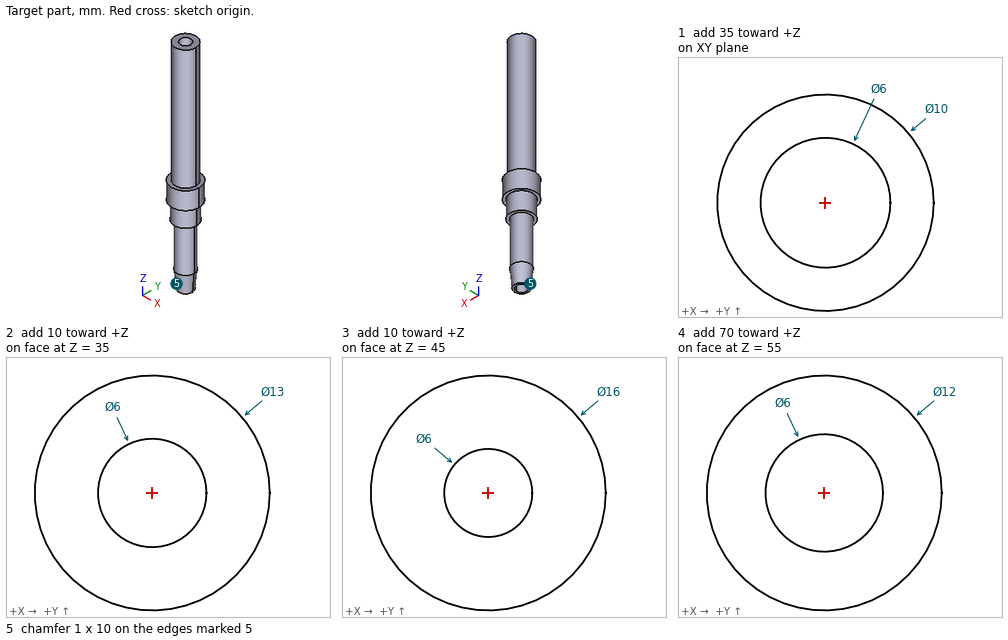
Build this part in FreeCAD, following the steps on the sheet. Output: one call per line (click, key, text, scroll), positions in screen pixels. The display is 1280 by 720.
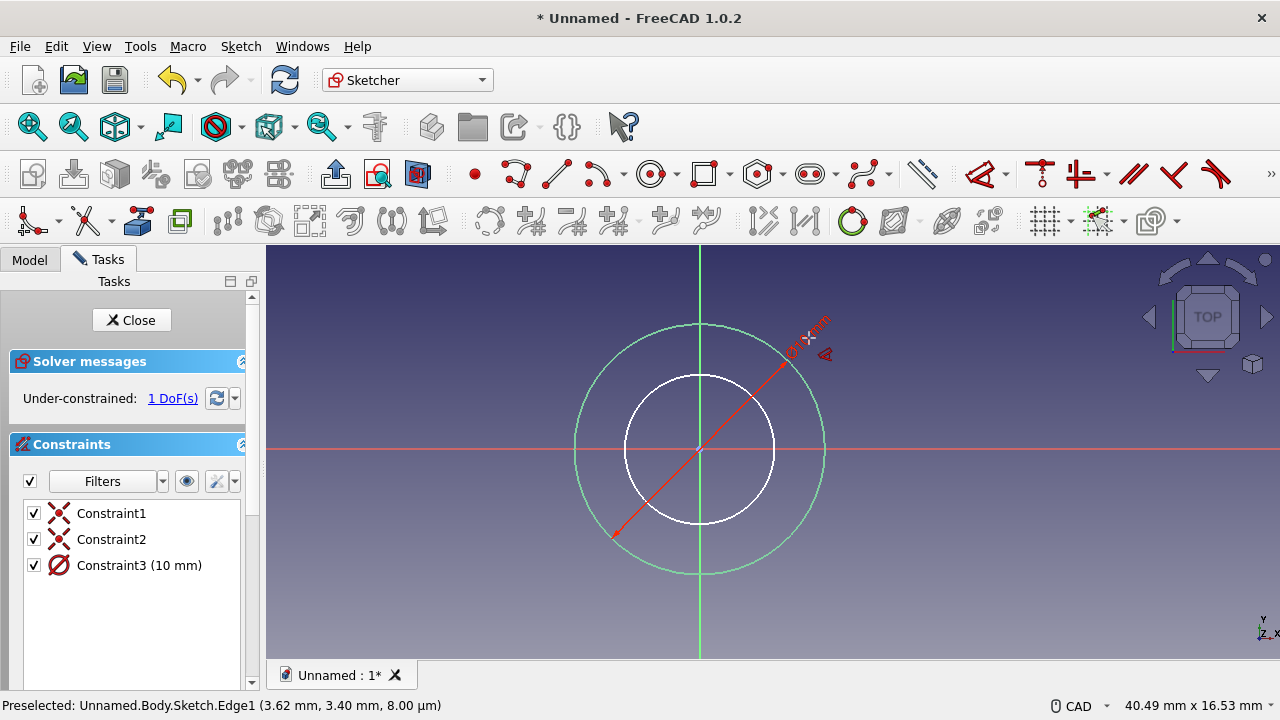
click(752, 396)
click(774, 373)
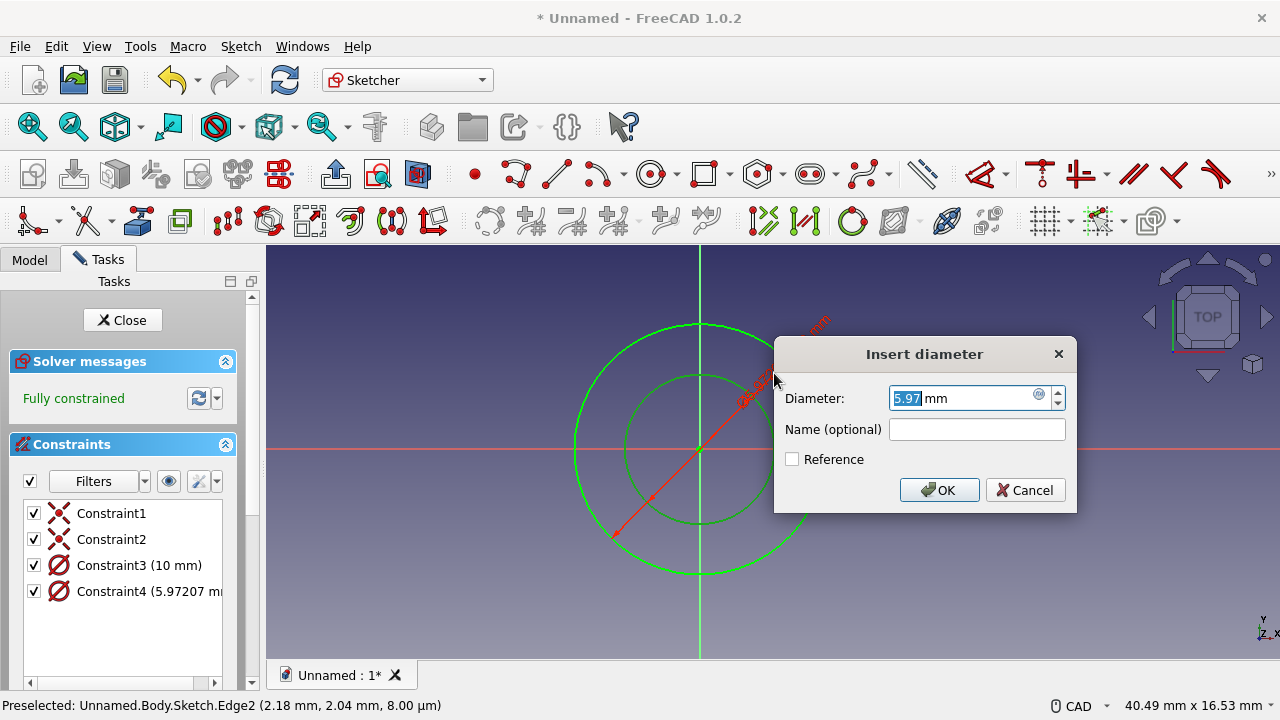
text(6)
key(Return)
key(Escape)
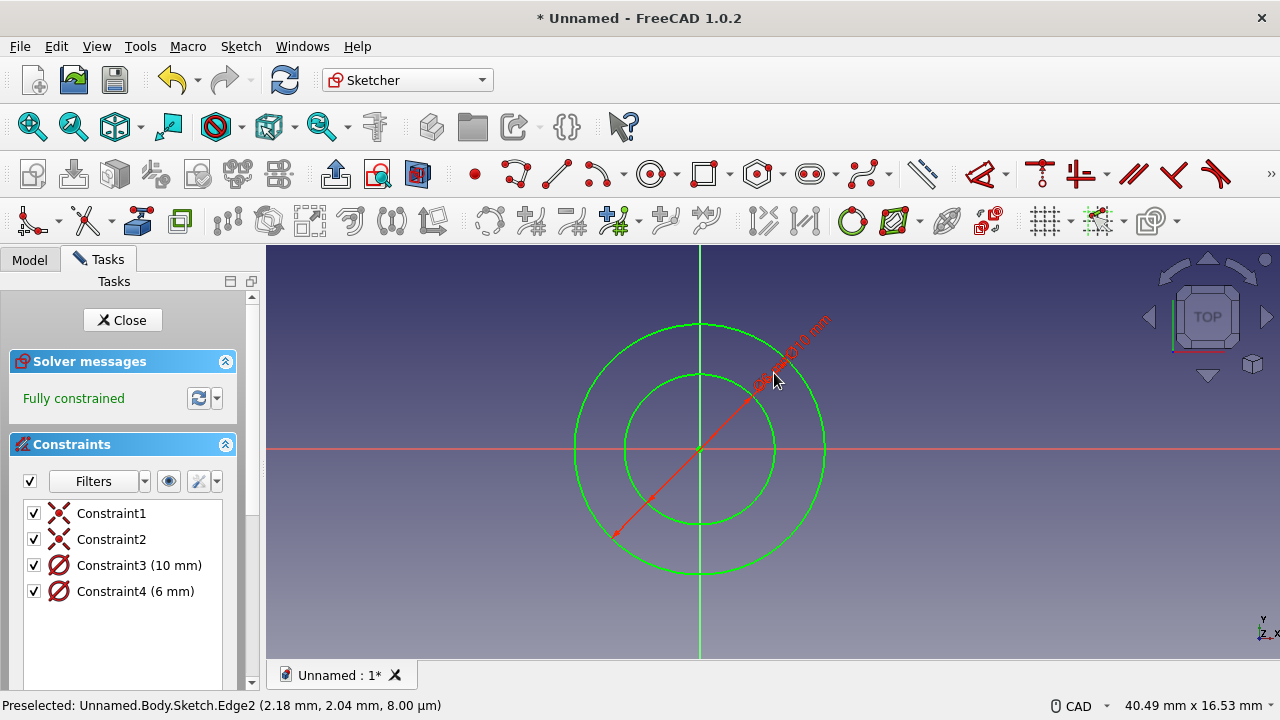
click(123, 320)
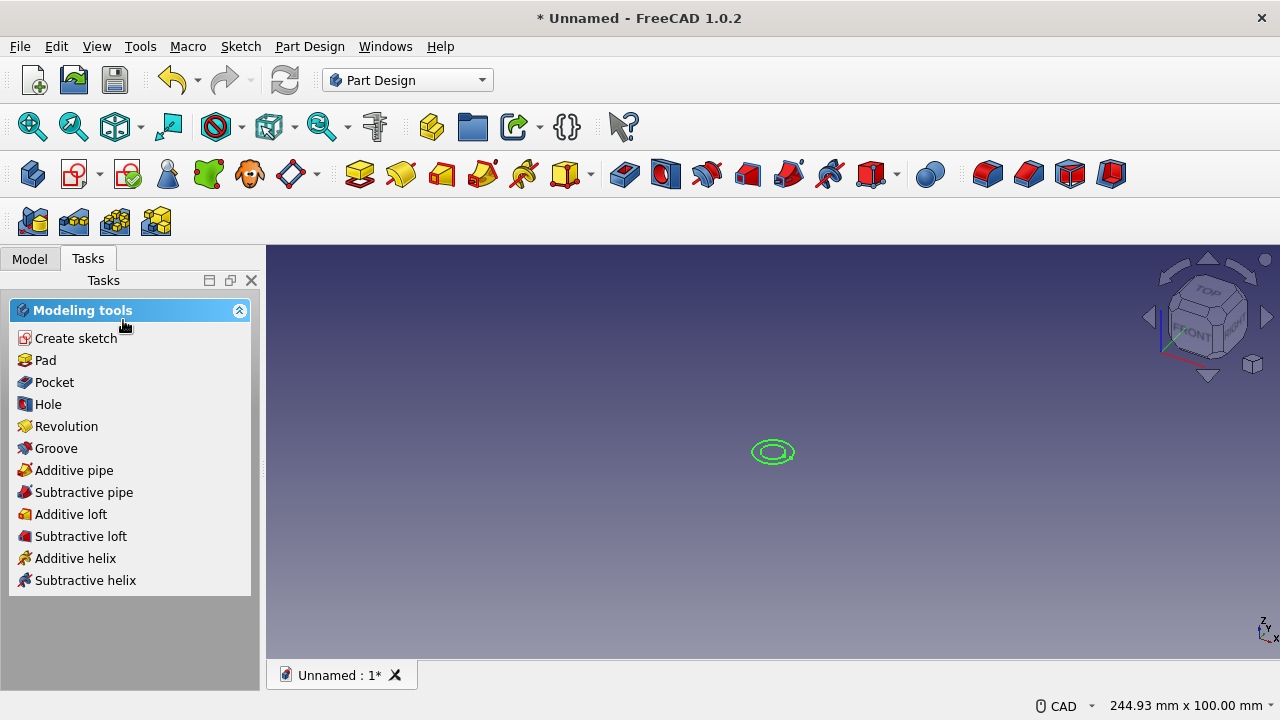
click(360, 174)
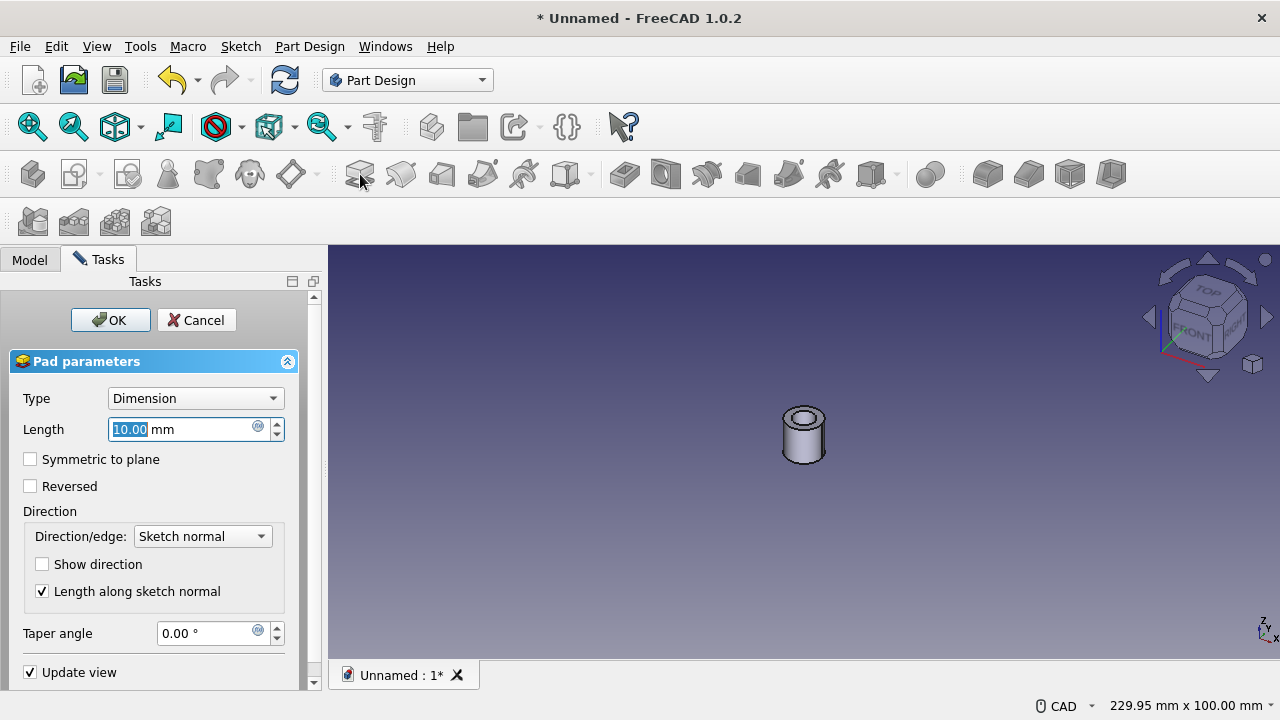
text(35)
key(Tab)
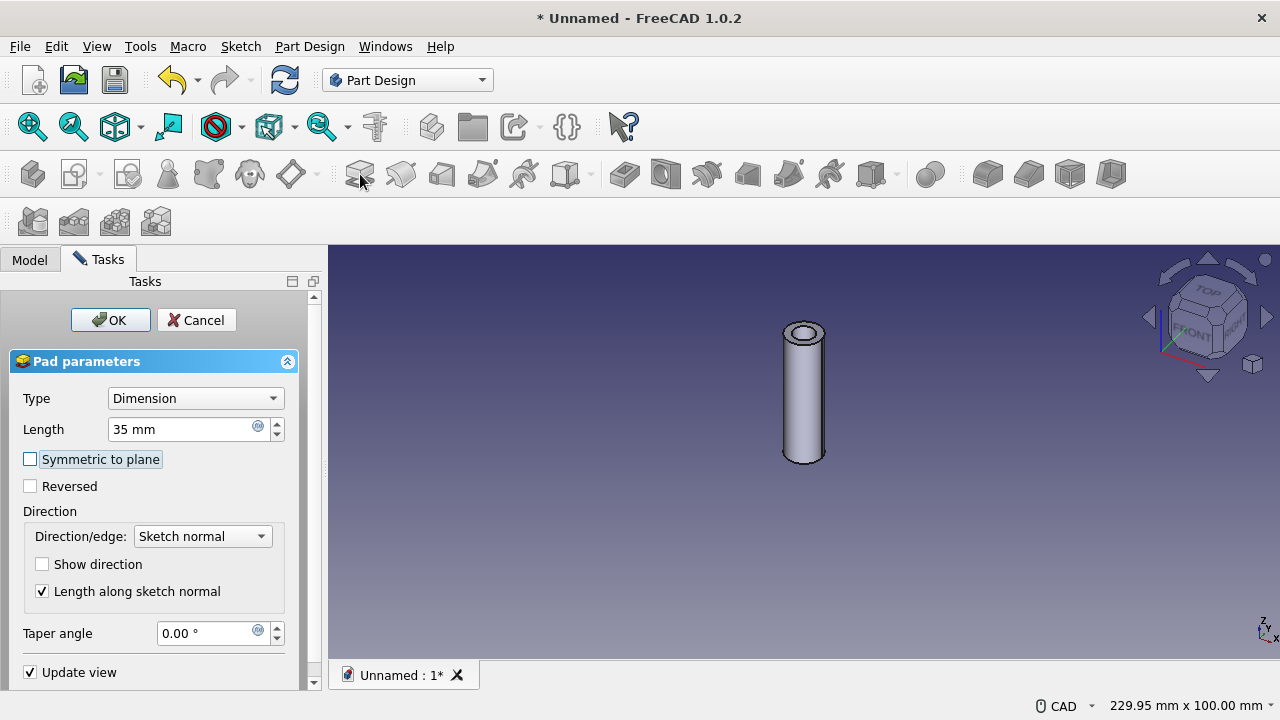
click(111, 320)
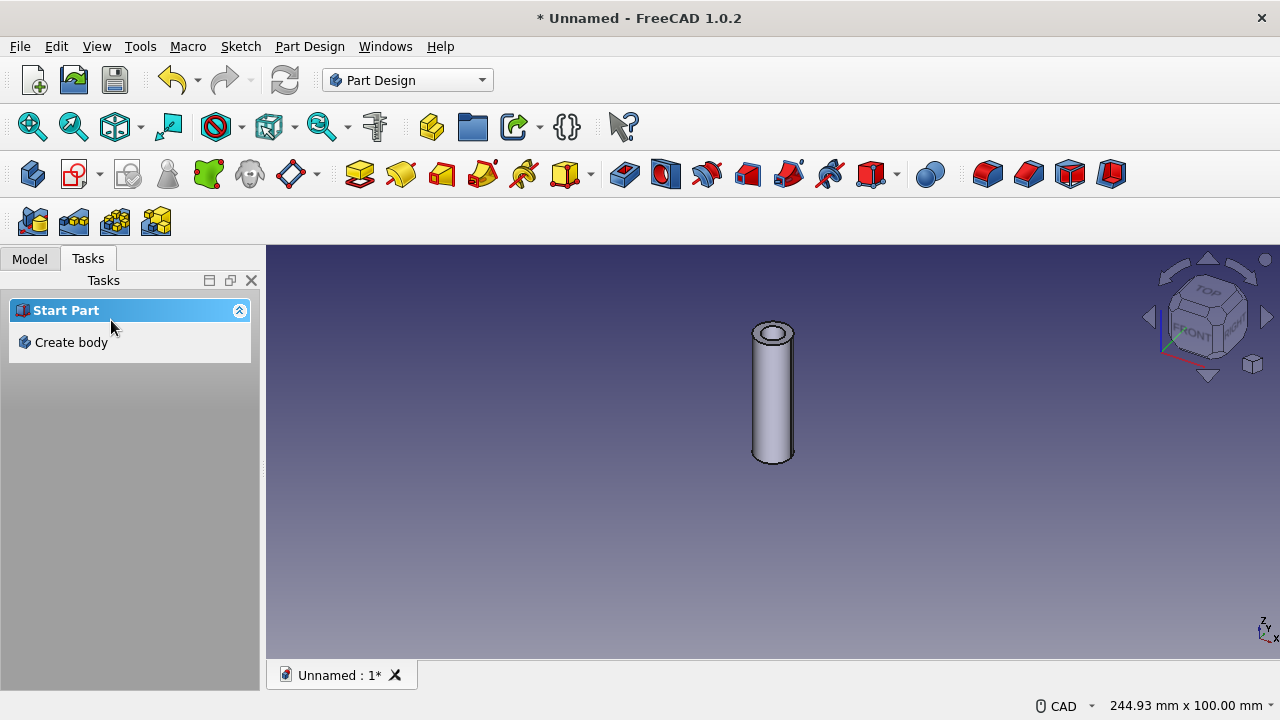
click(33, 128)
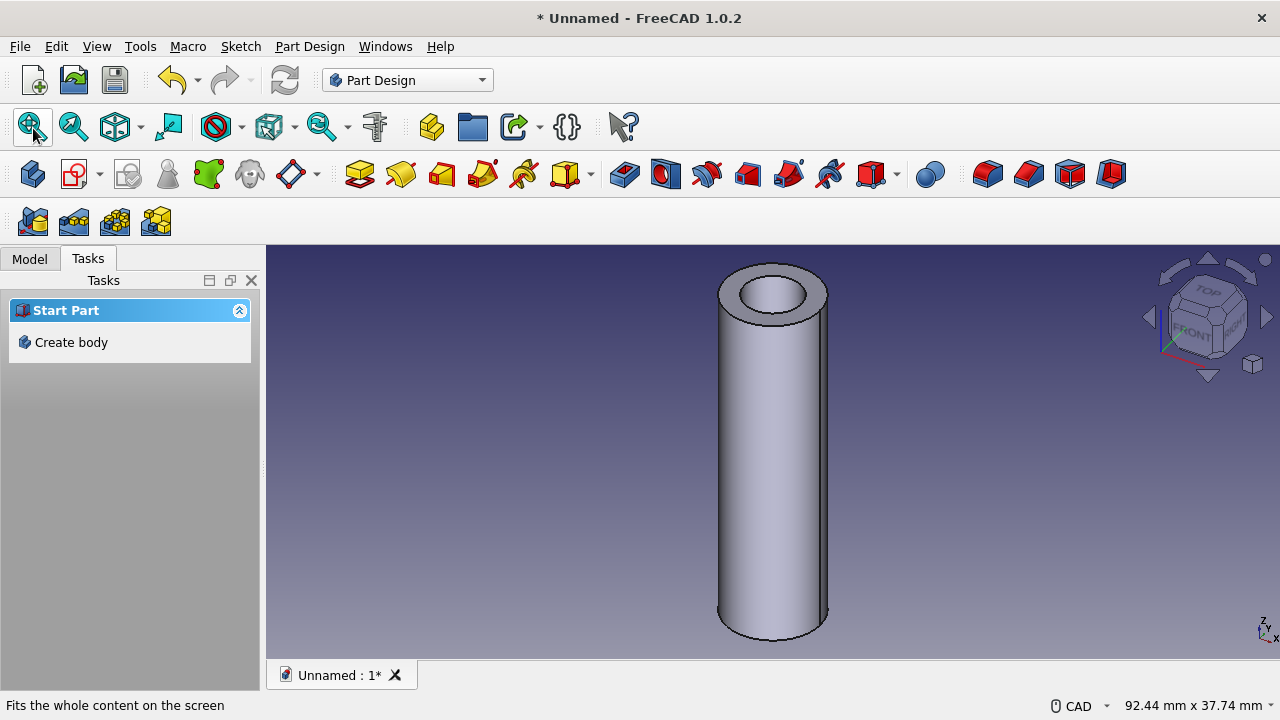
click(816, 287)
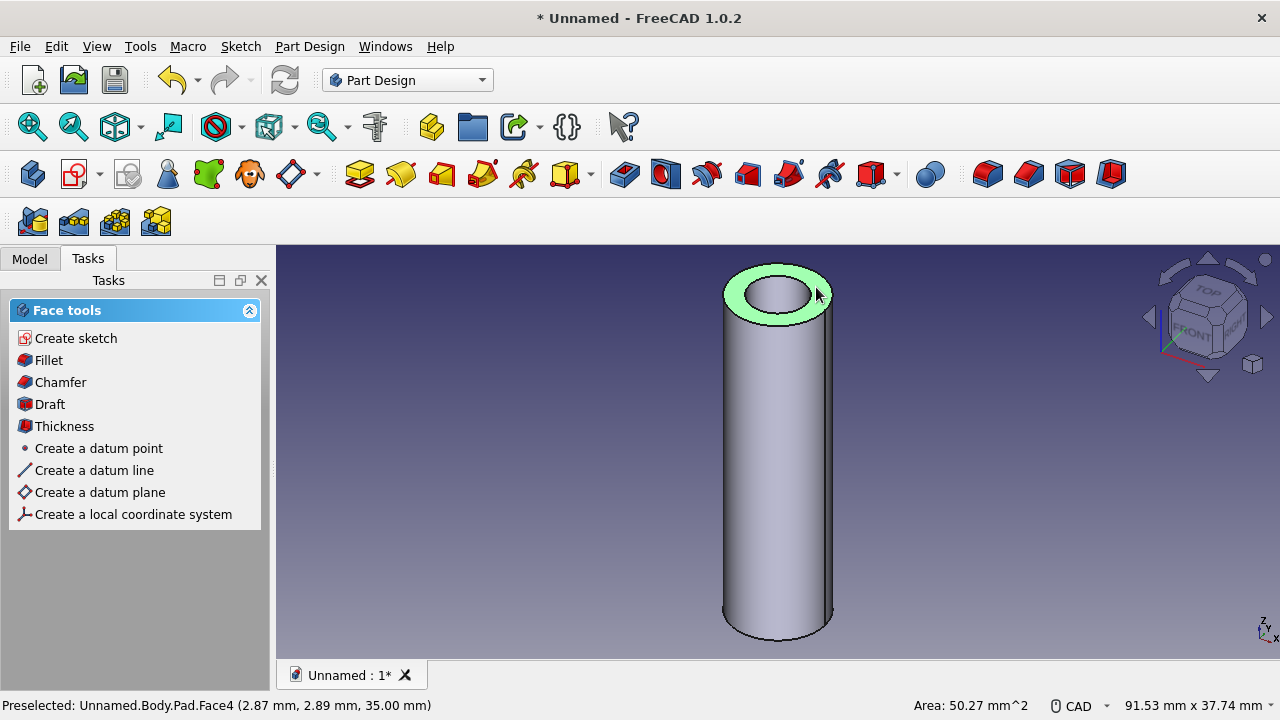
click(74, 174)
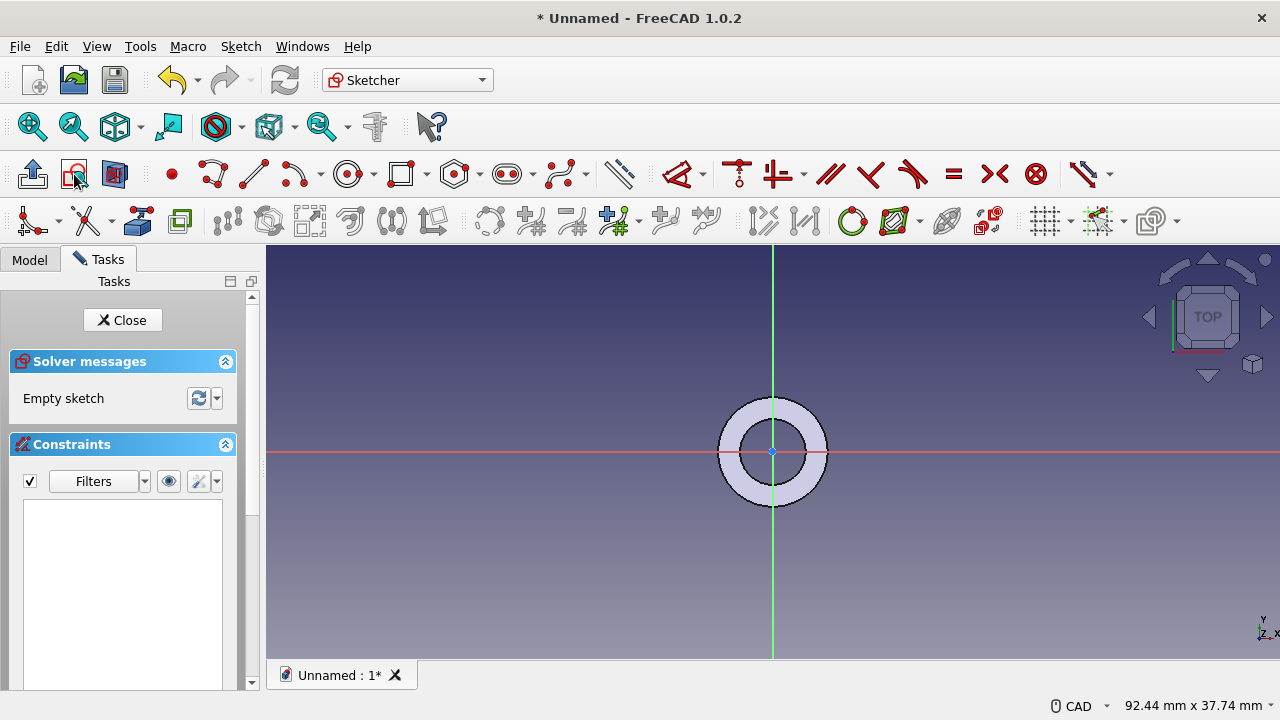
scroll(856, 452, up, 3)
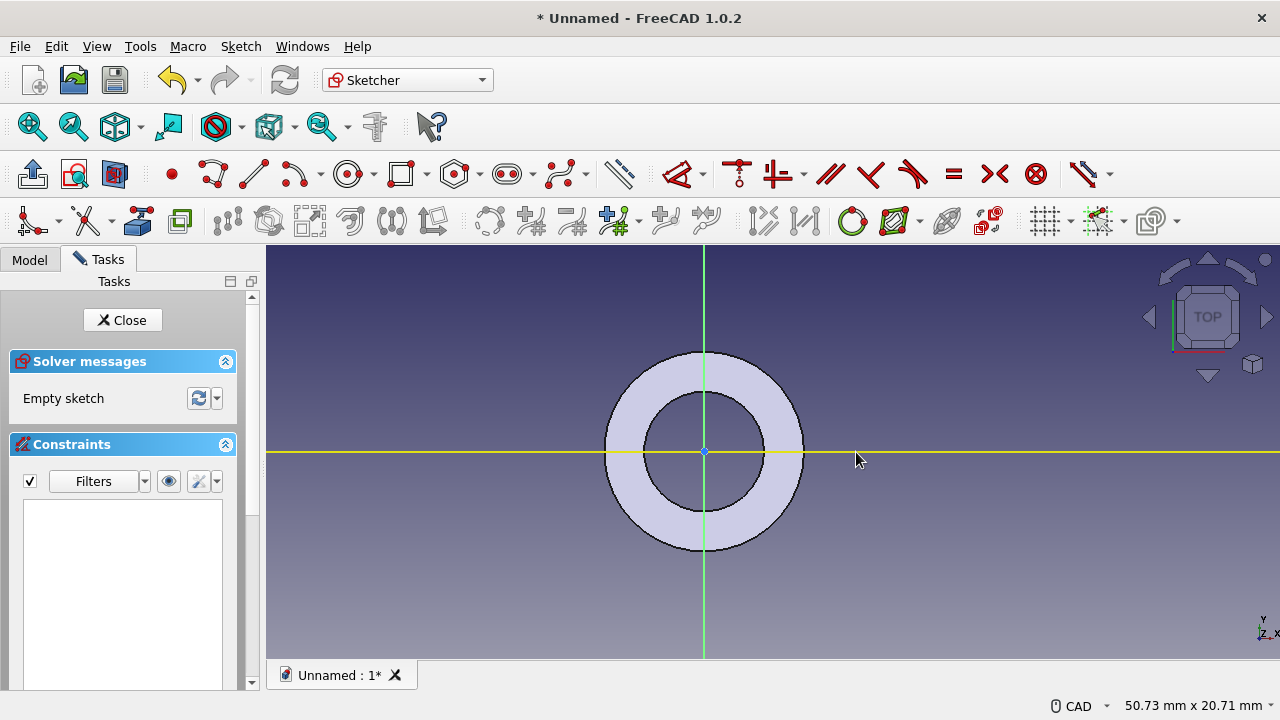
click(348, 174)